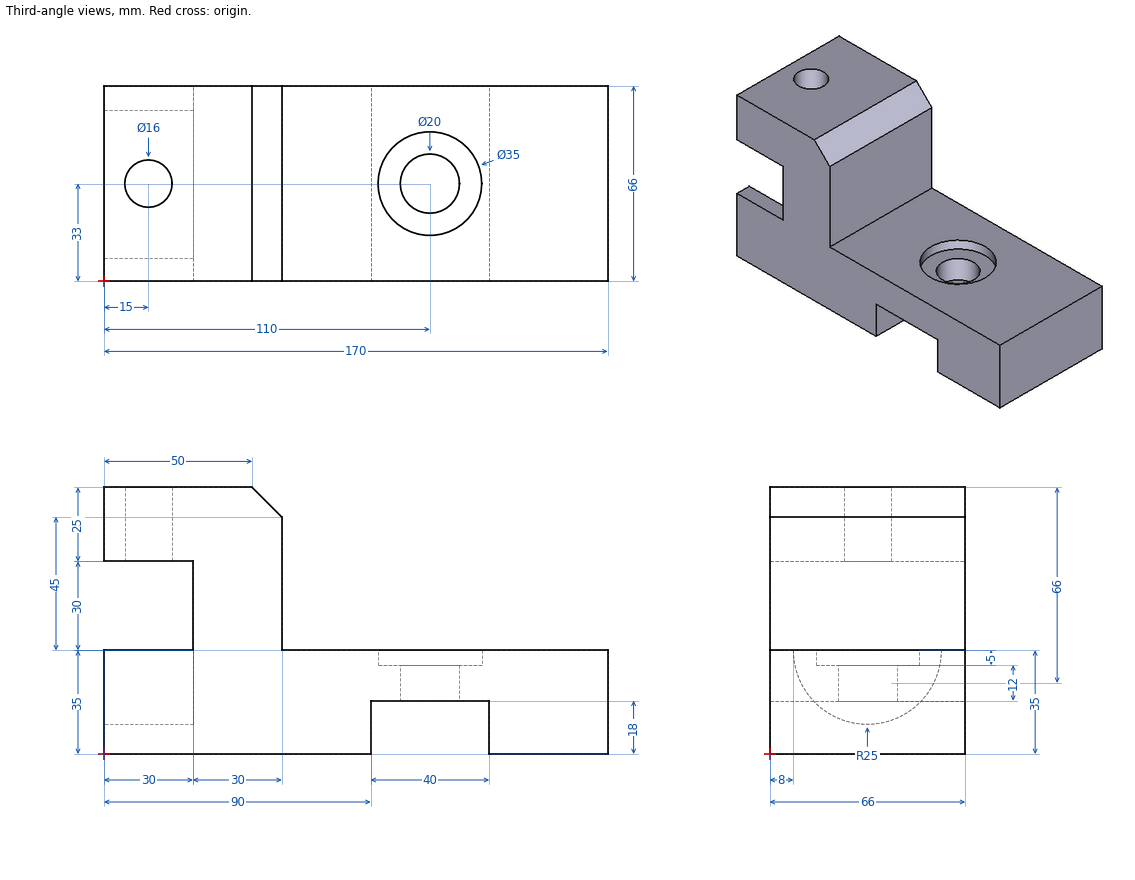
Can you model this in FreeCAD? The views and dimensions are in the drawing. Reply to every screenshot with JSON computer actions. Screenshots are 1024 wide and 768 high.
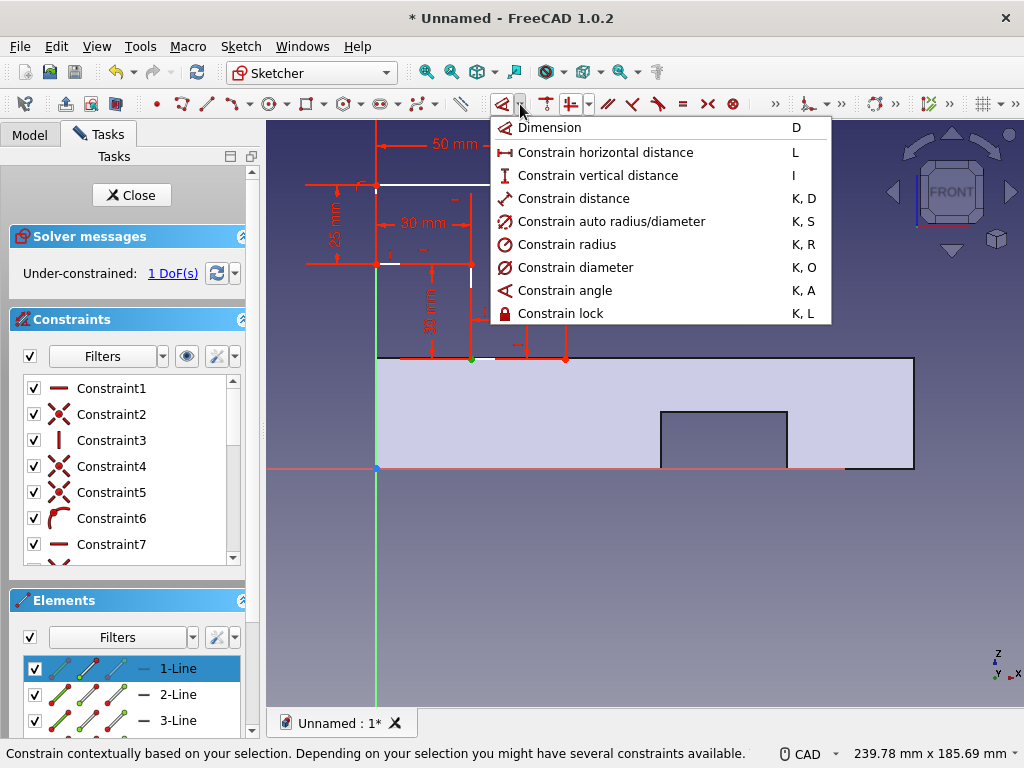
{"action": "left_click", "coordinate": [661, 176]}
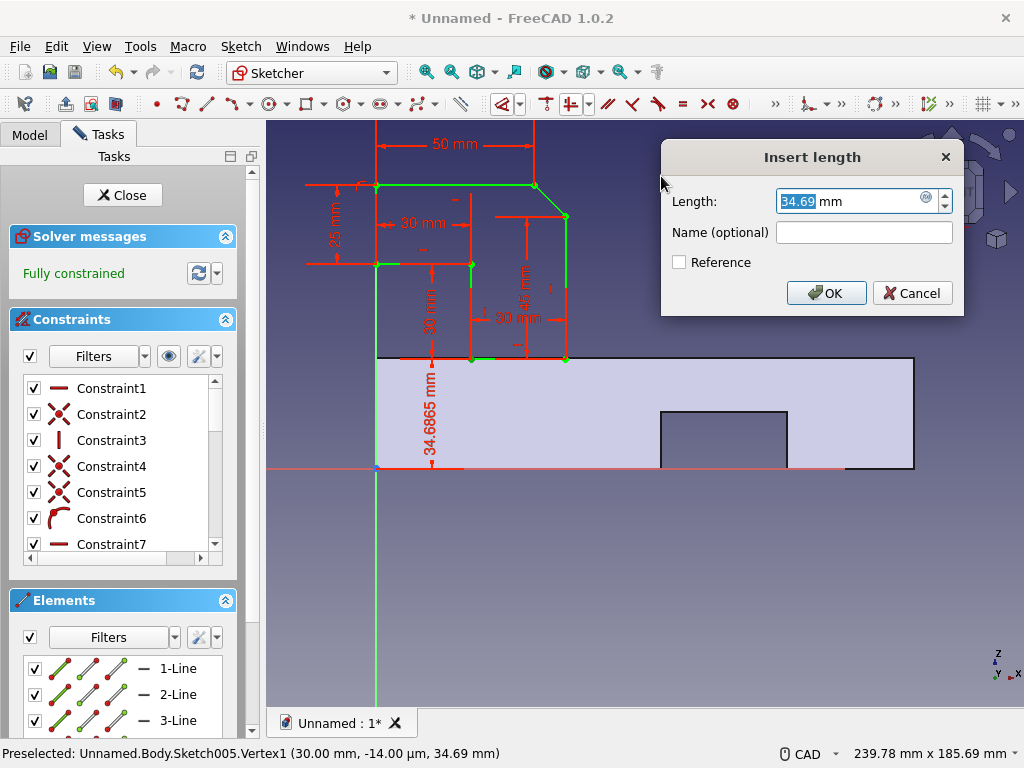
{"action": "type", "text": "35"}
{"action": "key", "text": "Return"}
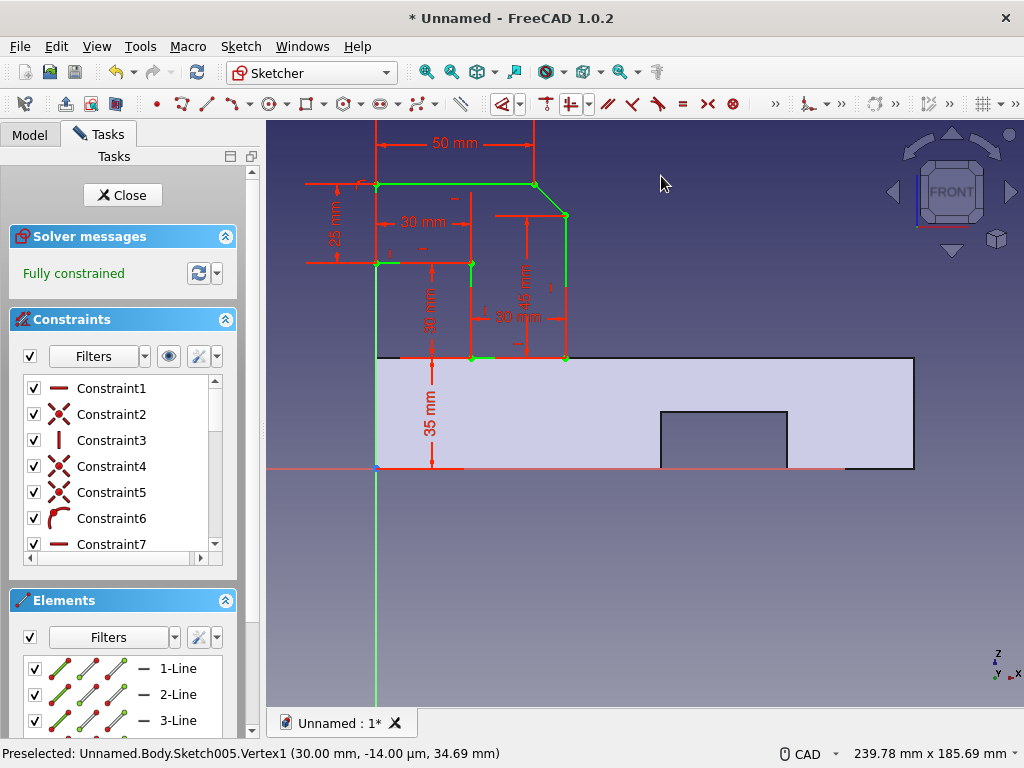
{"action": "left_click", "coordinate": [123, 195]}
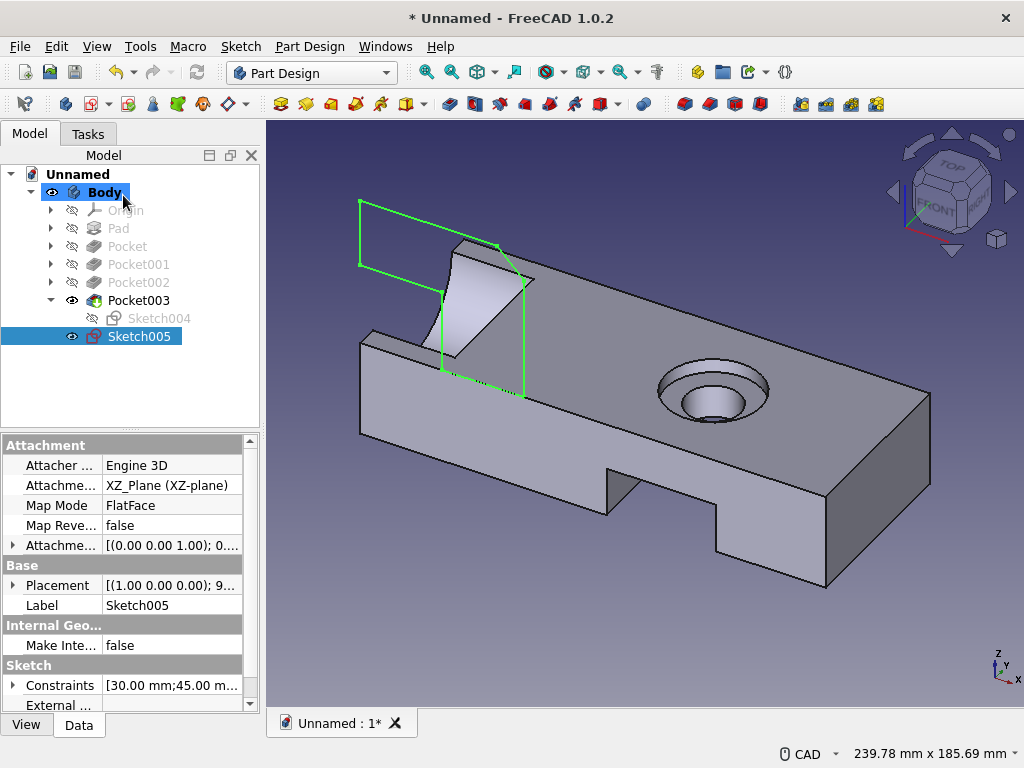
{"action": "left_click", "coordinate": [281, 104]}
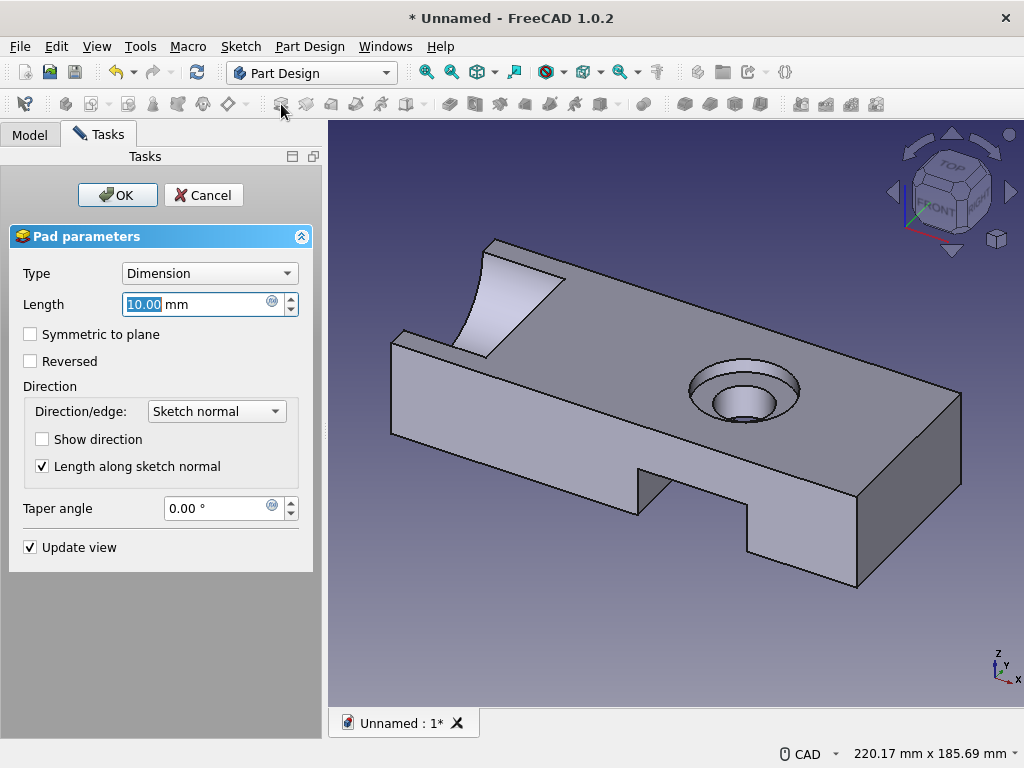
{"action": "type", "text": "66"}
{"action": "key", "text": "Tab"}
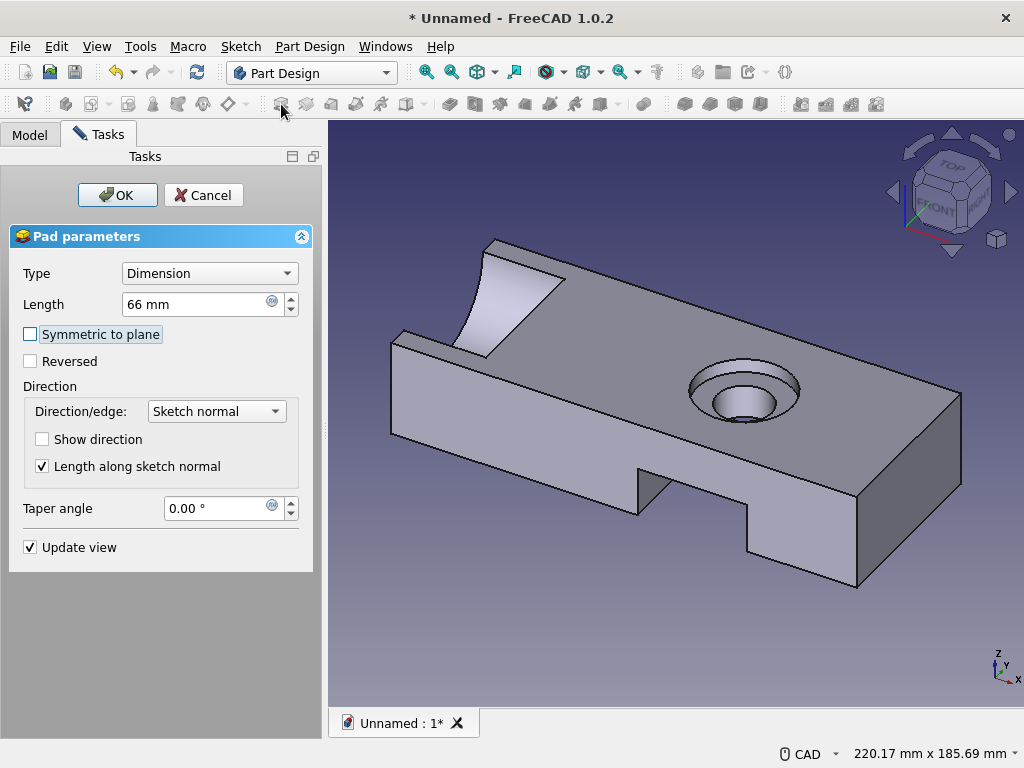
{"action": "left_click", "coordinate": [31, 361]}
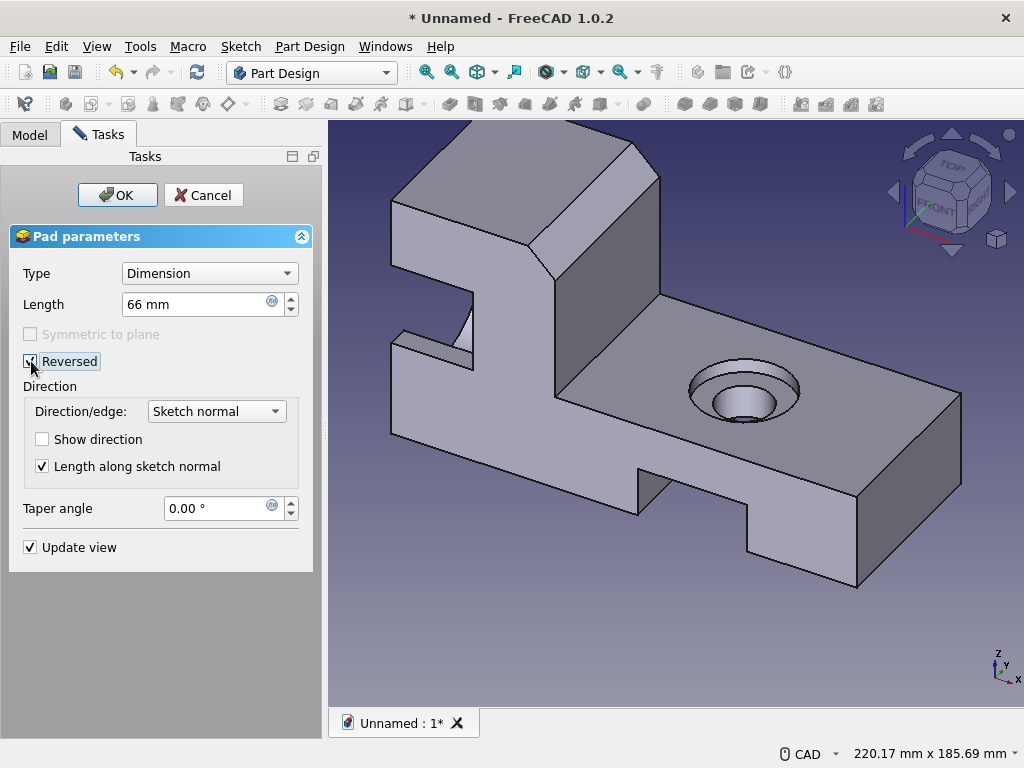
{"action": "left_click", "coordinate": [118, 195]}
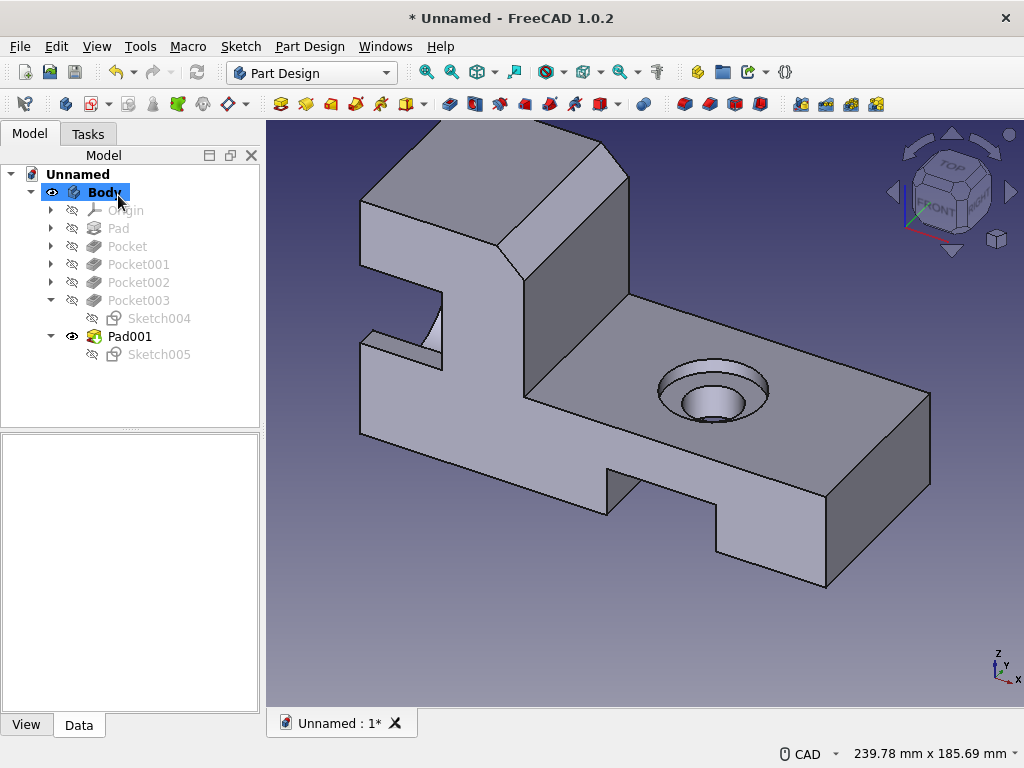
{"action": "key", "text": "v f"}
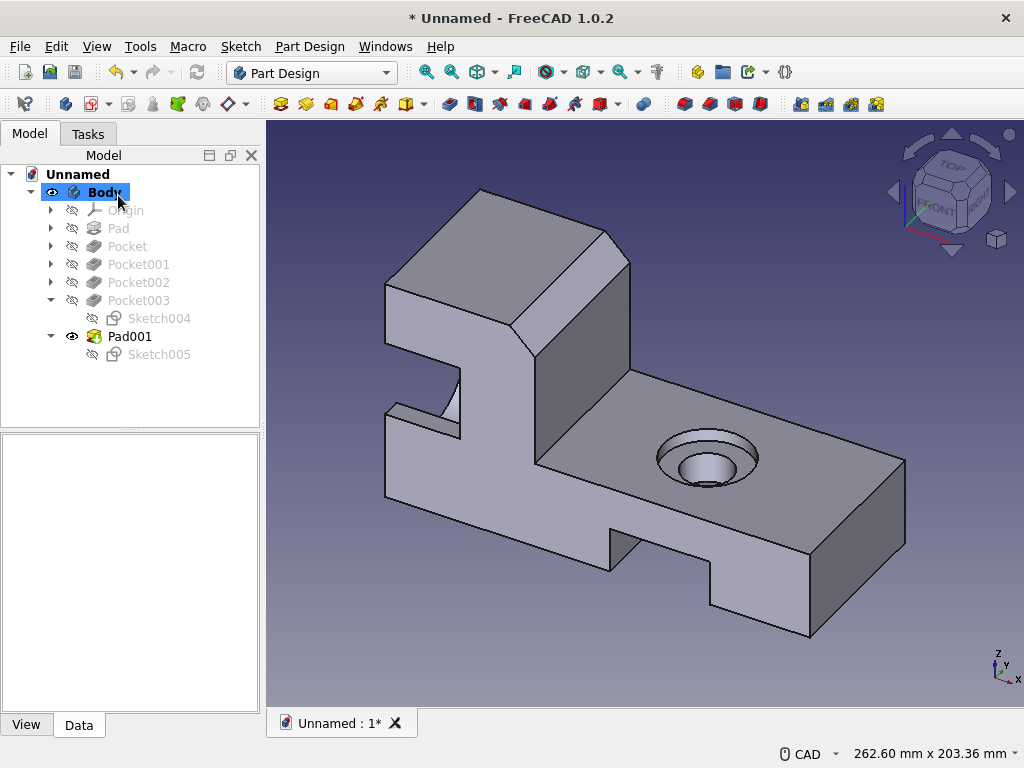
{"action": "left_click", "coordinate": [495, 256]}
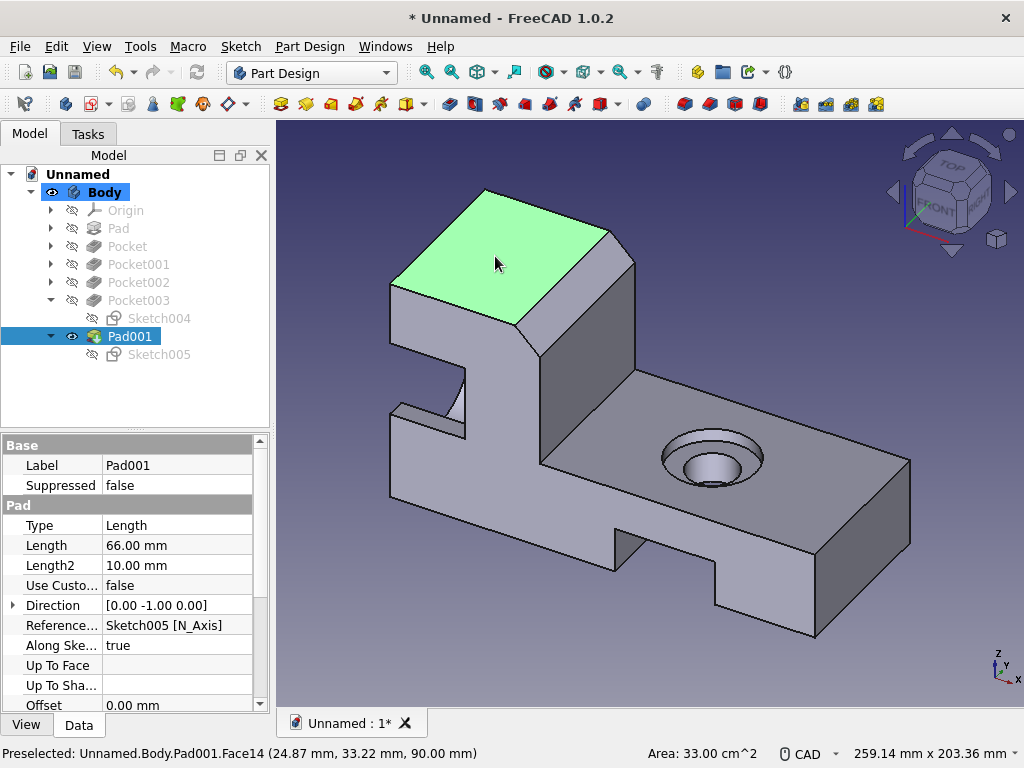
{"action": "left_click", "coordinate": [90, 104]}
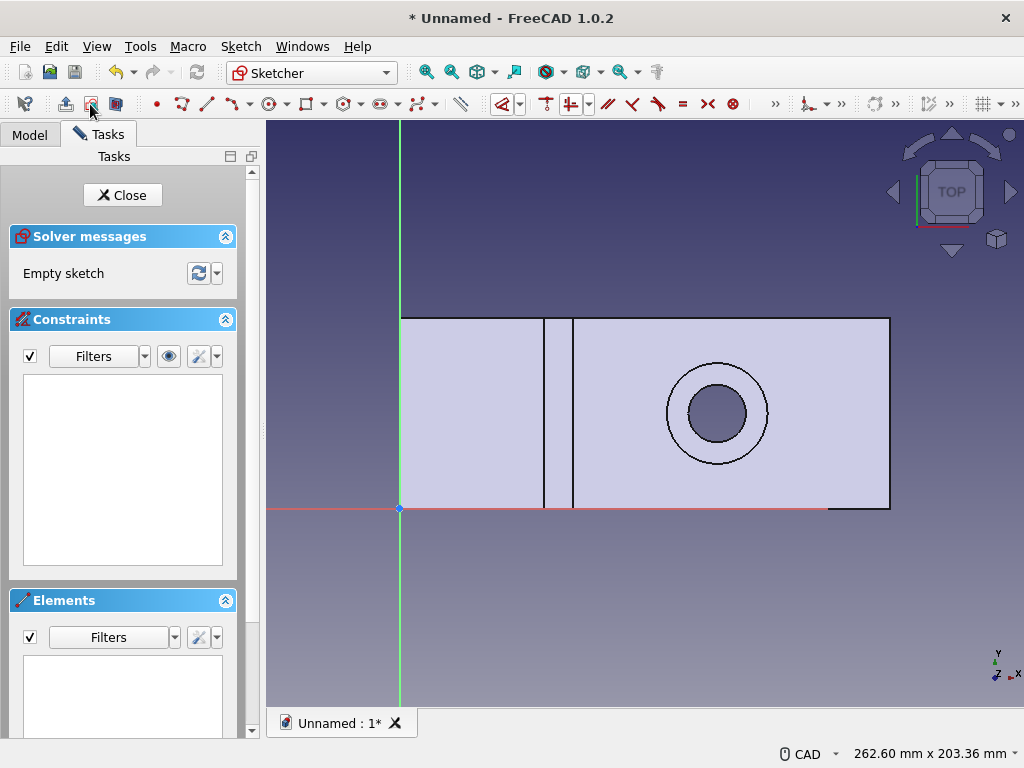
{"action": "scroll", "coordinate": [422, 413], "scroll_direction": "up", "scroll_amount": 10}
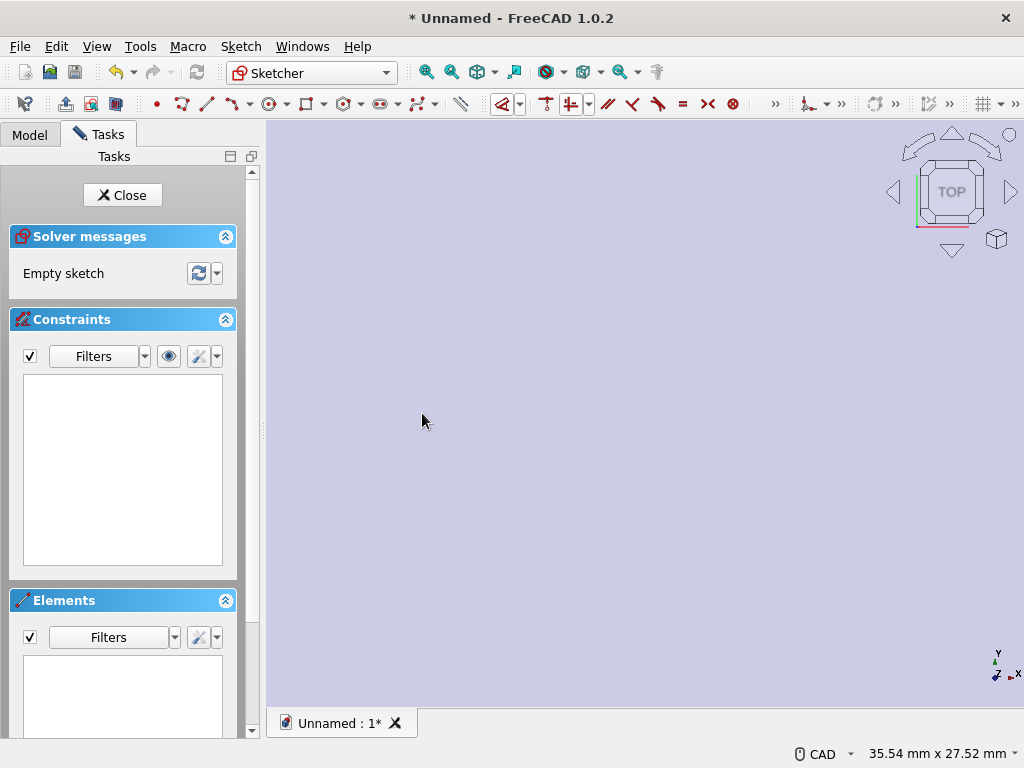
{"action": "key", "text": "g c"}